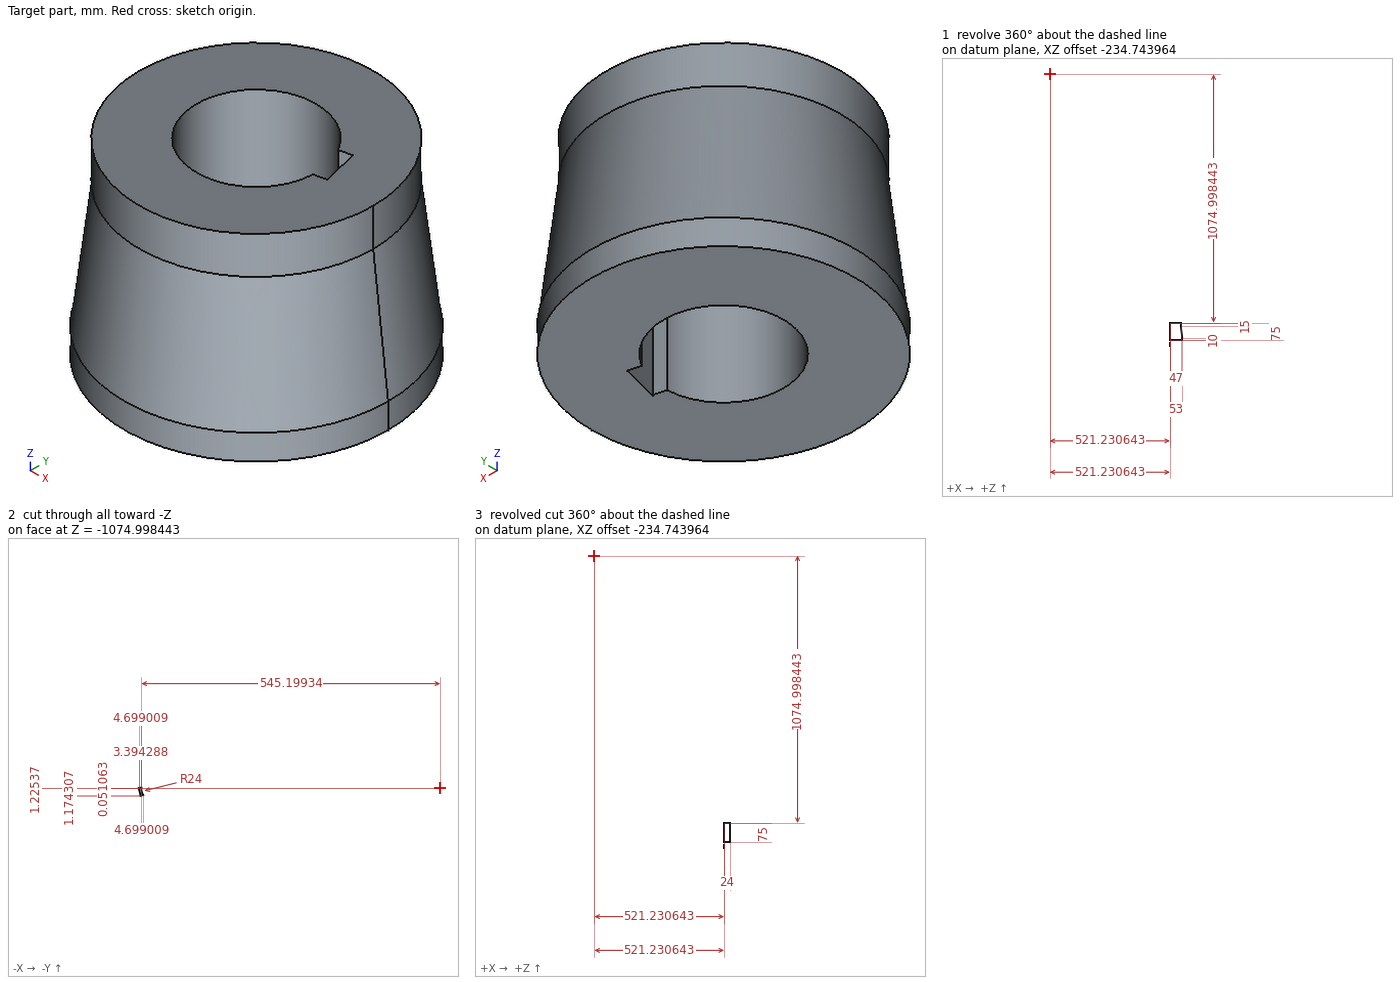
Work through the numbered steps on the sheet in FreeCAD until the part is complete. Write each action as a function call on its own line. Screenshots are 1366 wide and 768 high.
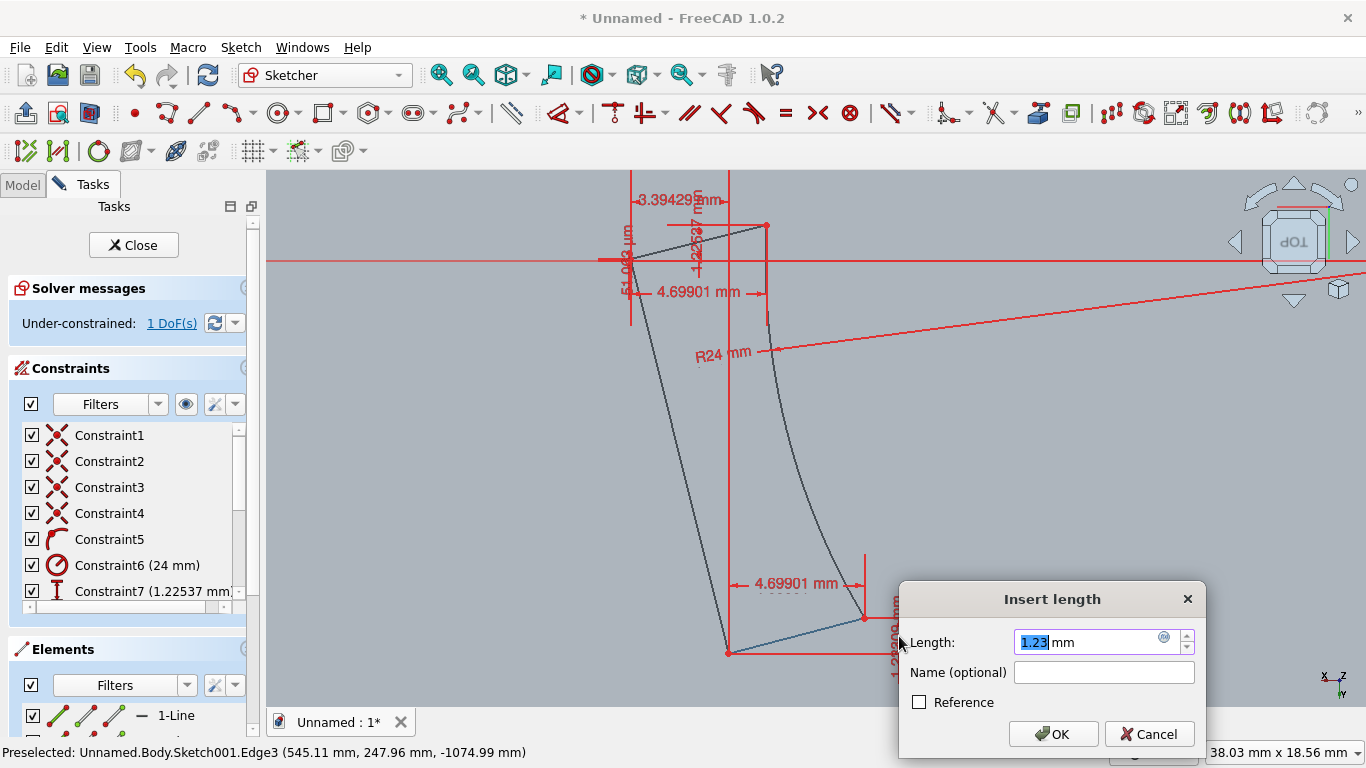
text(1.174307)
key(Return)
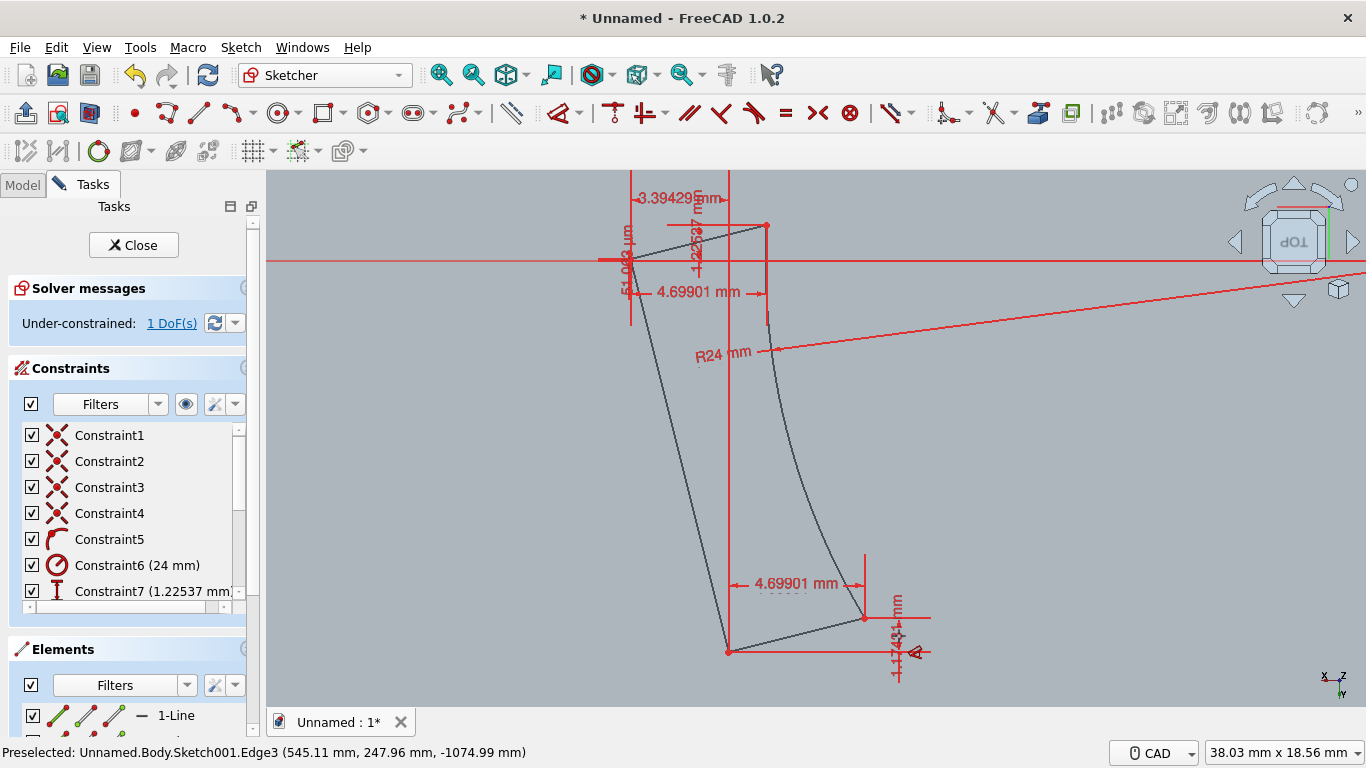
click(767, 225)
click(984, 295)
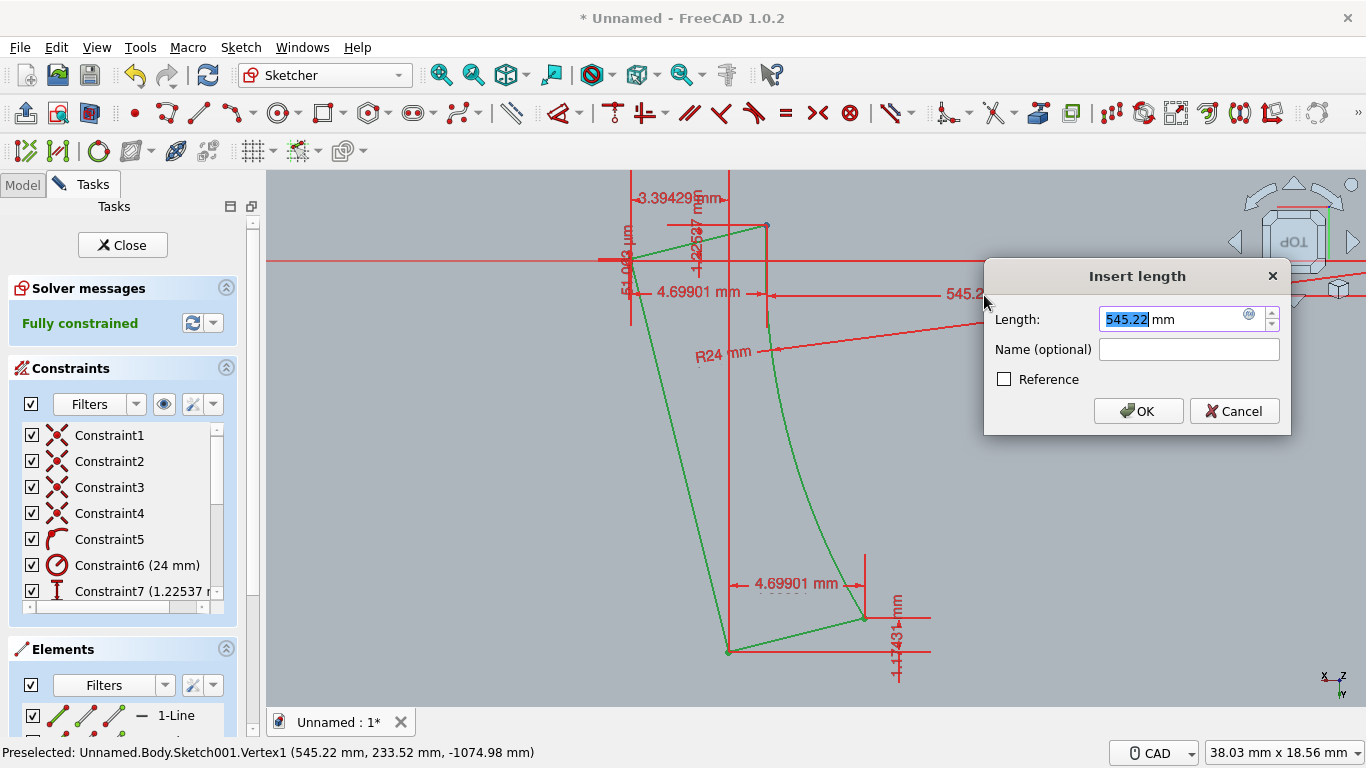
text(545.19934)
key(Return)
key(Escape)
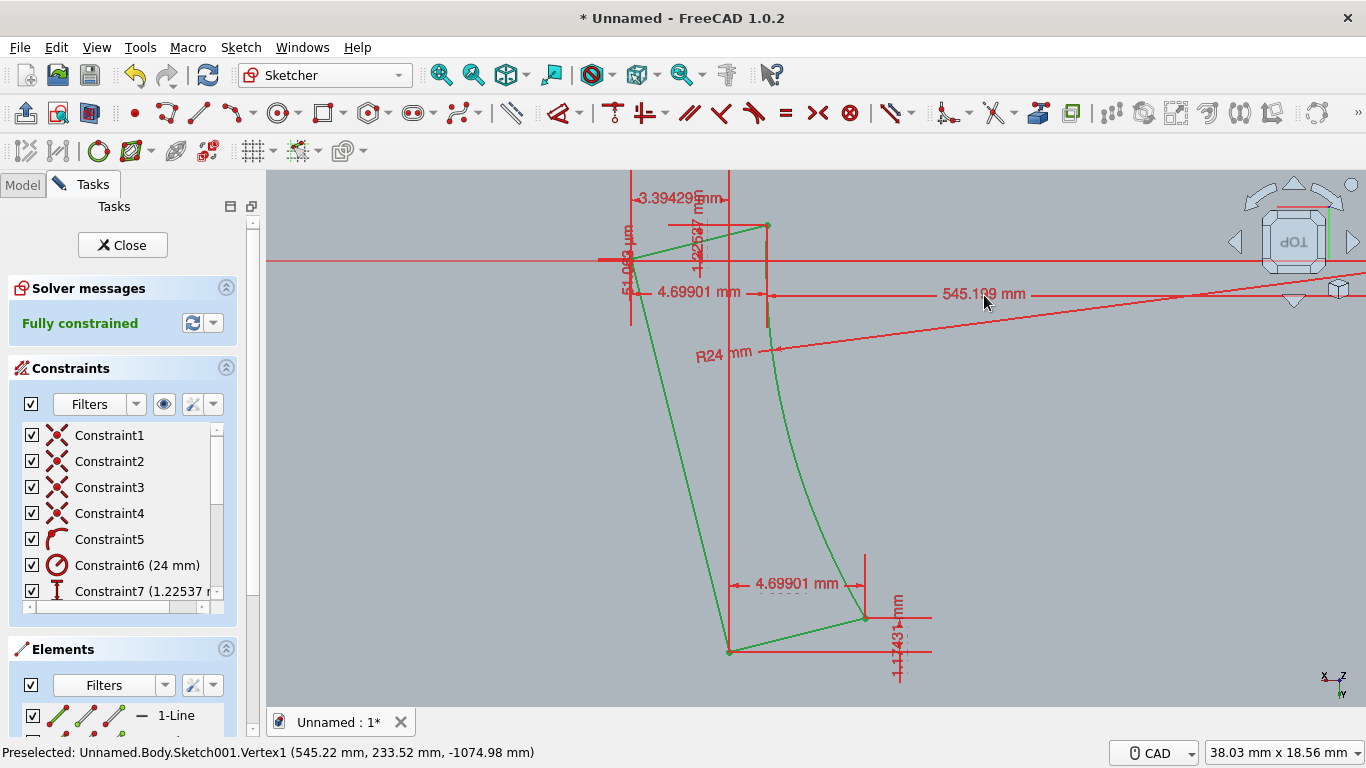
click(123, 245)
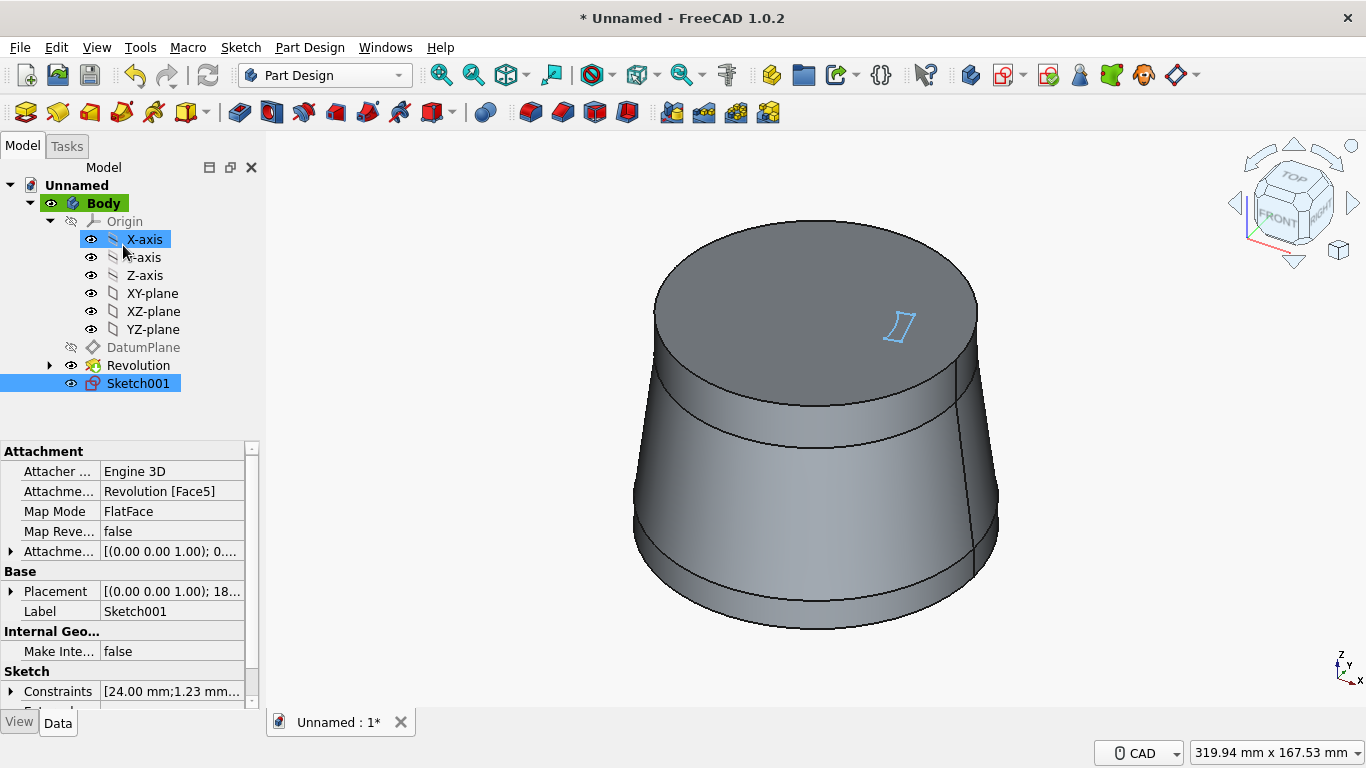
click(240, 112)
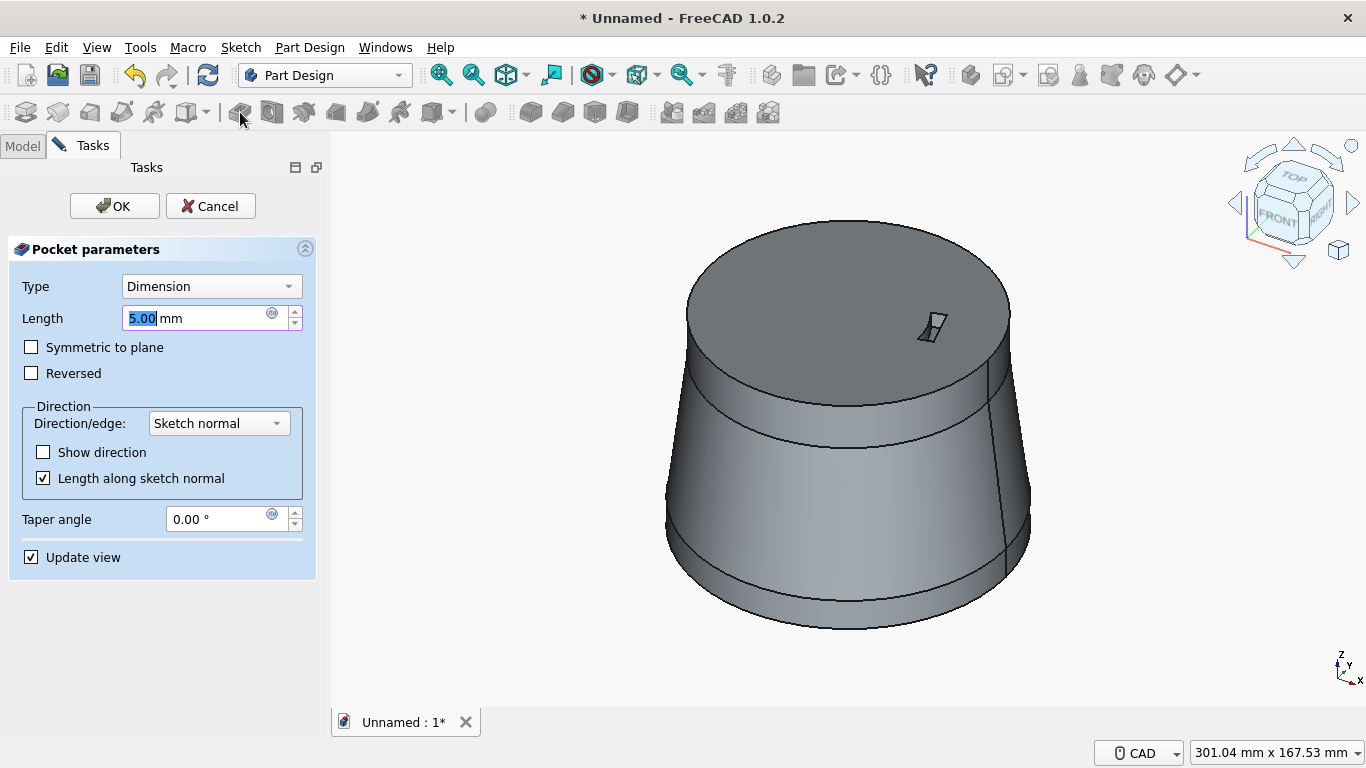
click(212, 286)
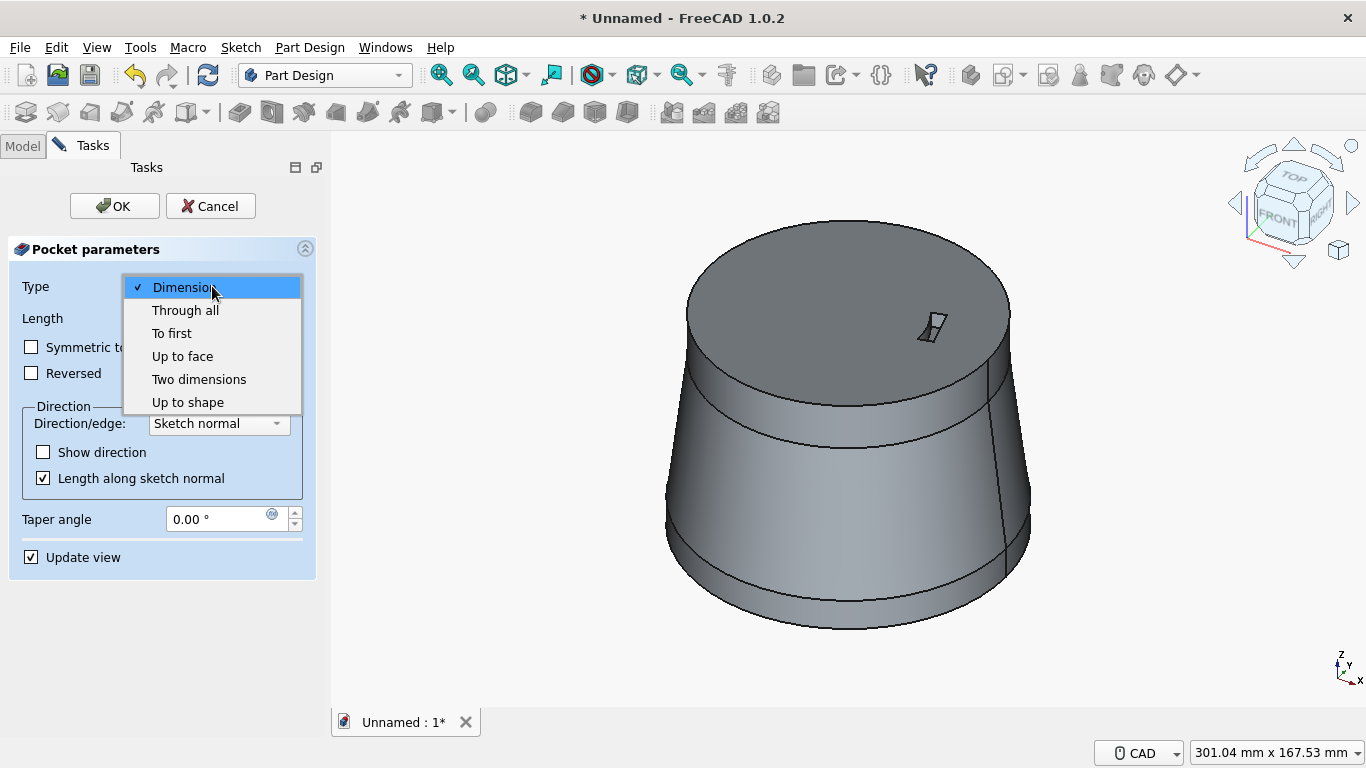
click(212, 310)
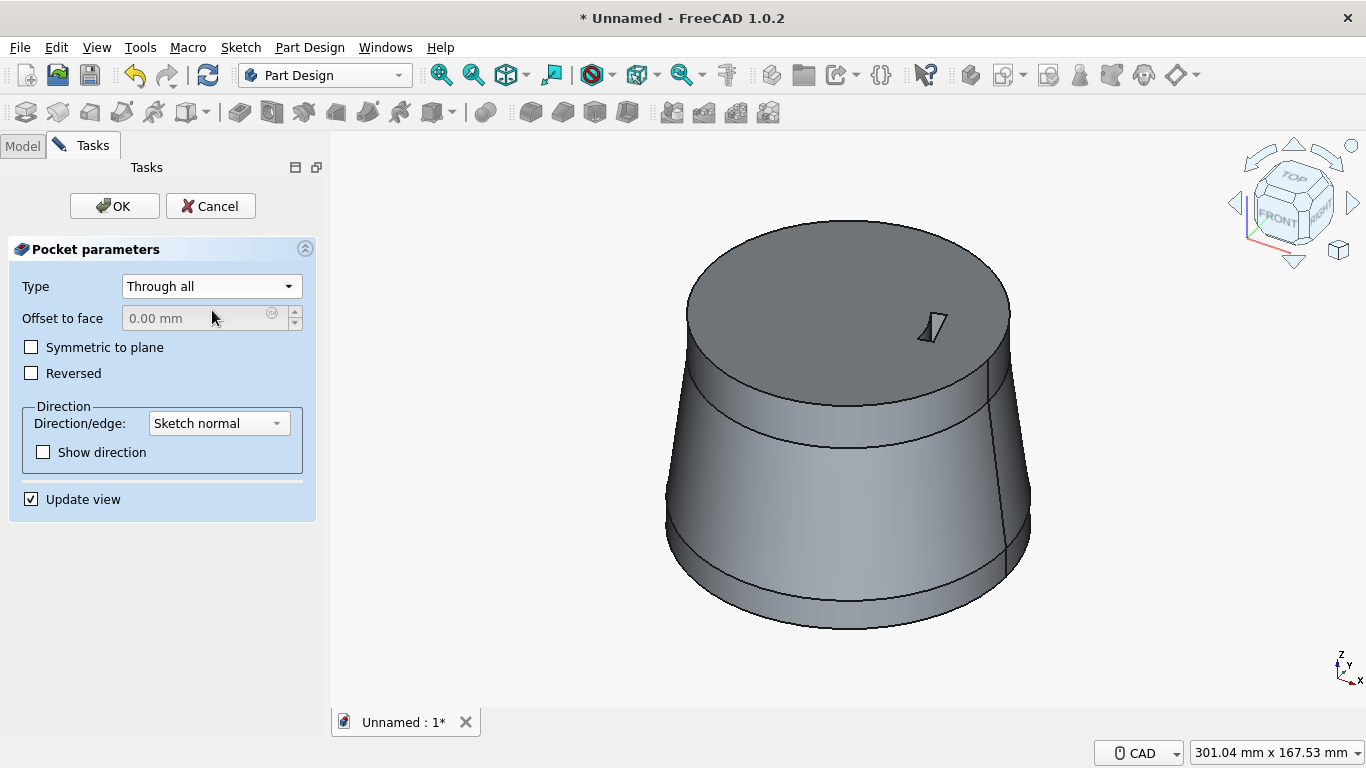
click(115, 206)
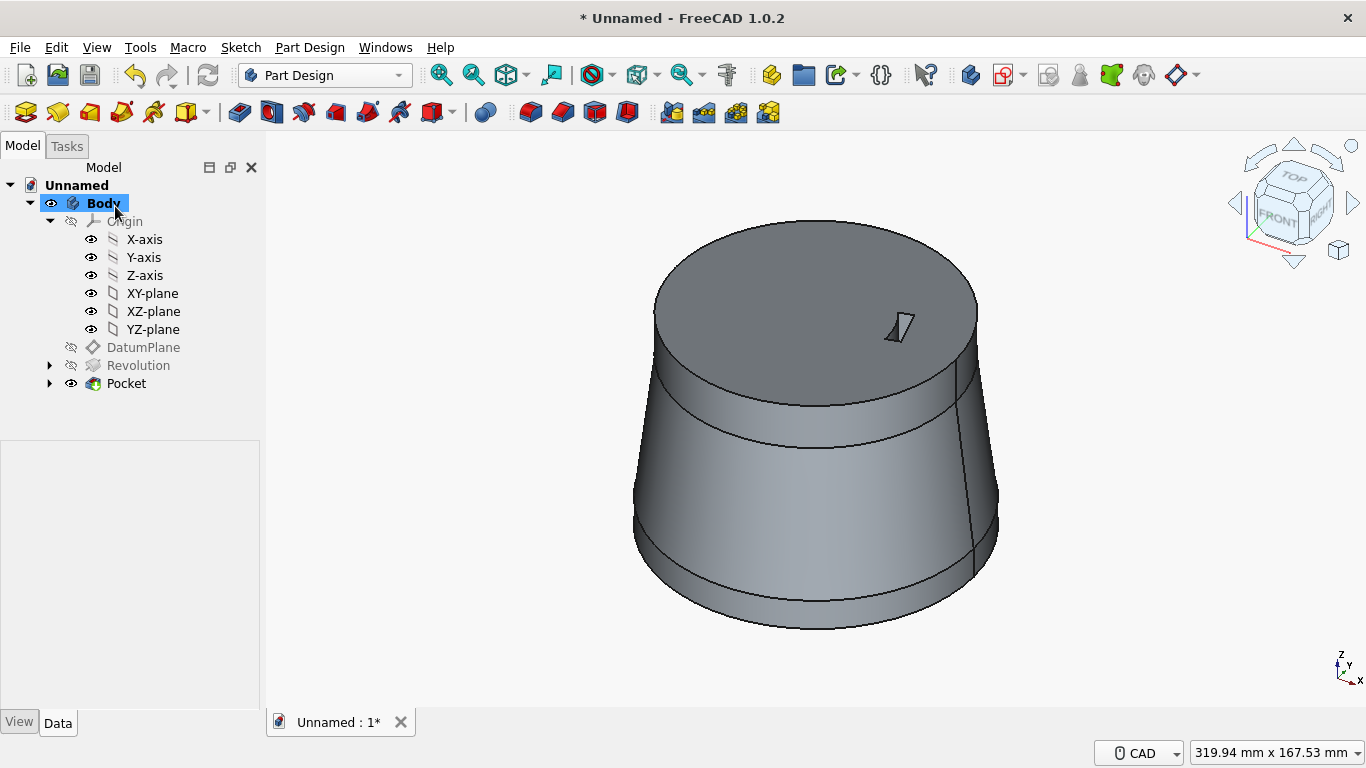
click(136, 311)